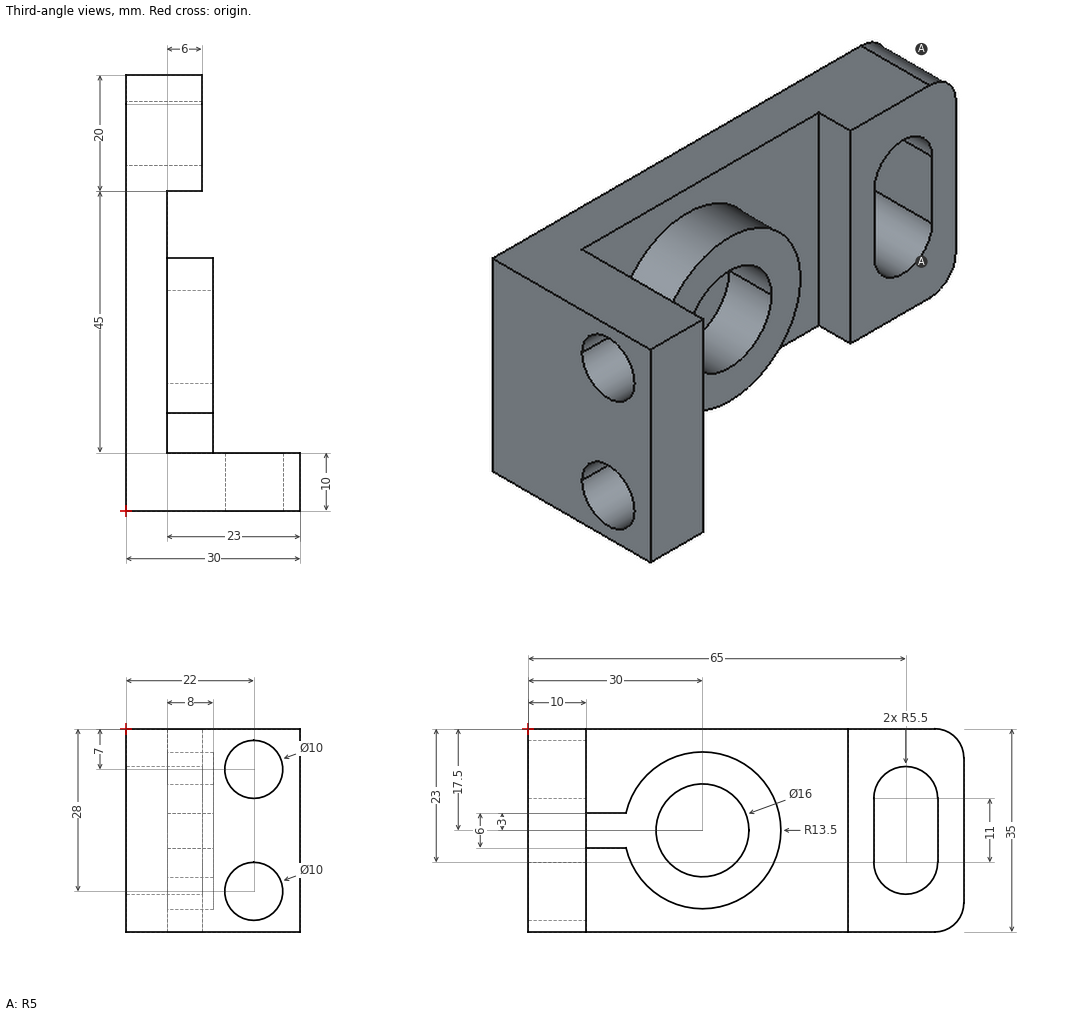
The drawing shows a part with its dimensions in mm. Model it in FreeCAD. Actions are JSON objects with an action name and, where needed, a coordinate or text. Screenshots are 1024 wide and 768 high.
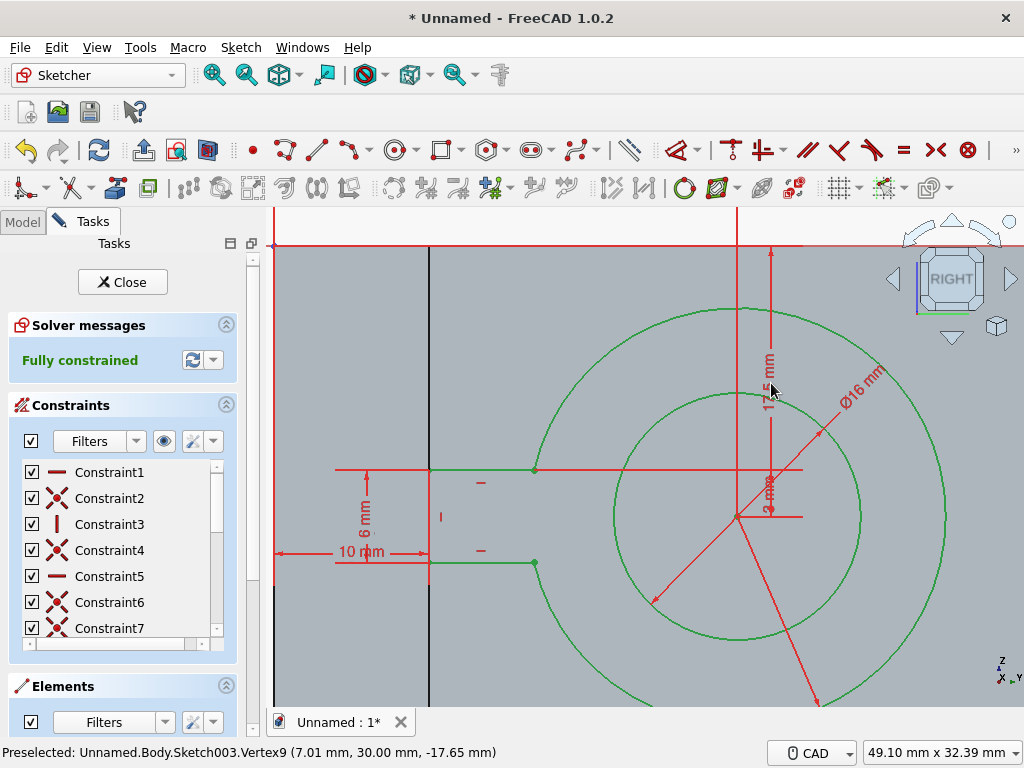
{"action": "left_click", "coordinate": [123, 282]}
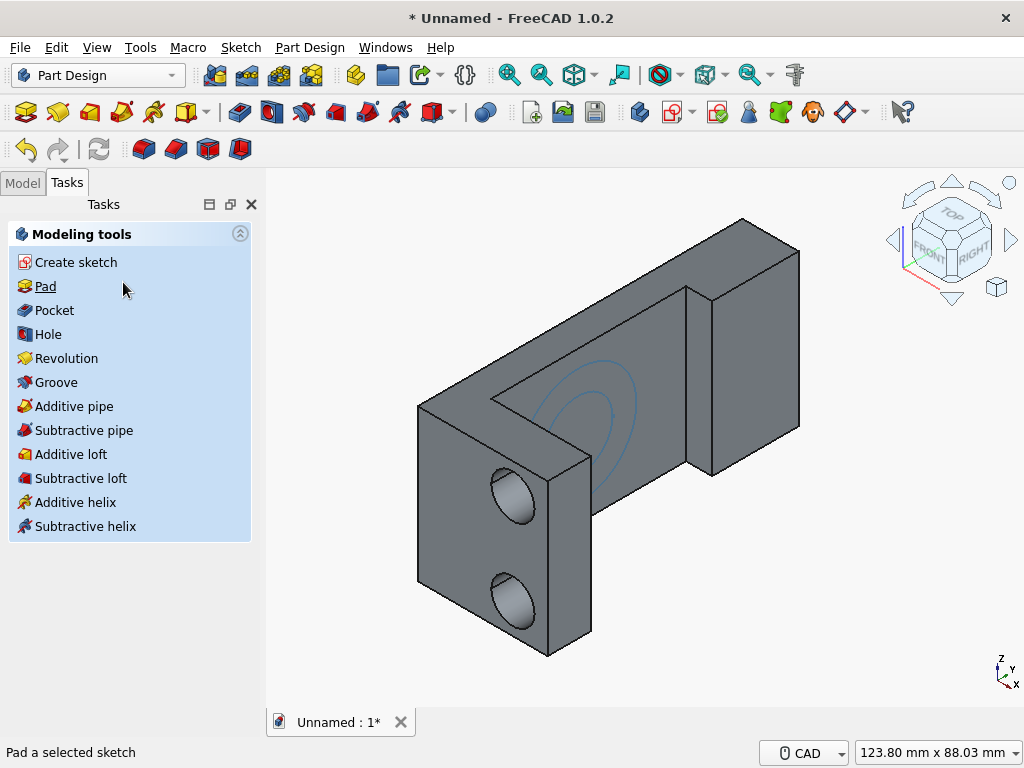
{"action": "left_click", "coordinate": [26, 112]}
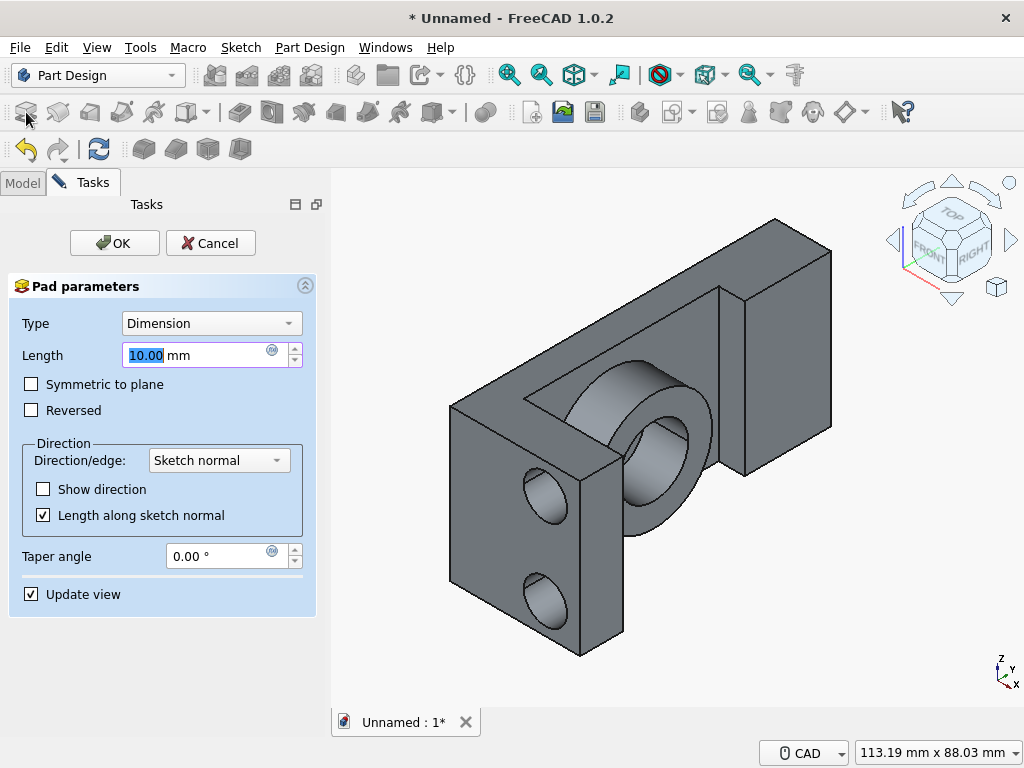
{"action": "type", "text": "8"}
{"action": "key", "text": "Tab"}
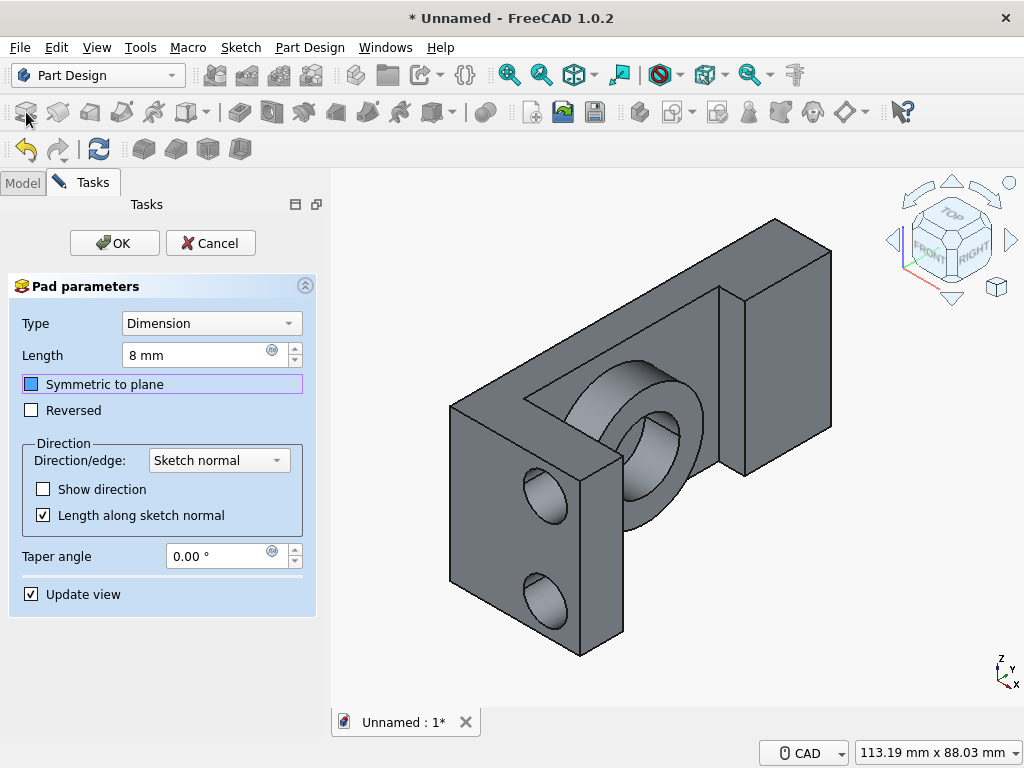
{"action": "left_click", "coordinate": [115, 243]}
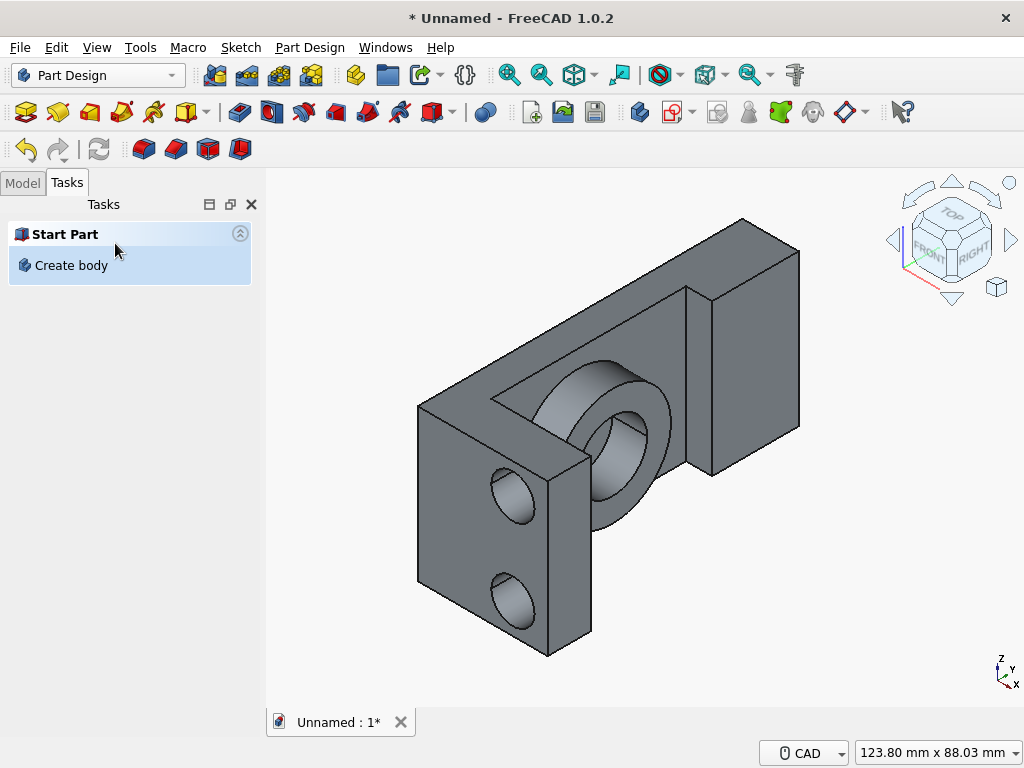
{"action": "key", "text": "2"}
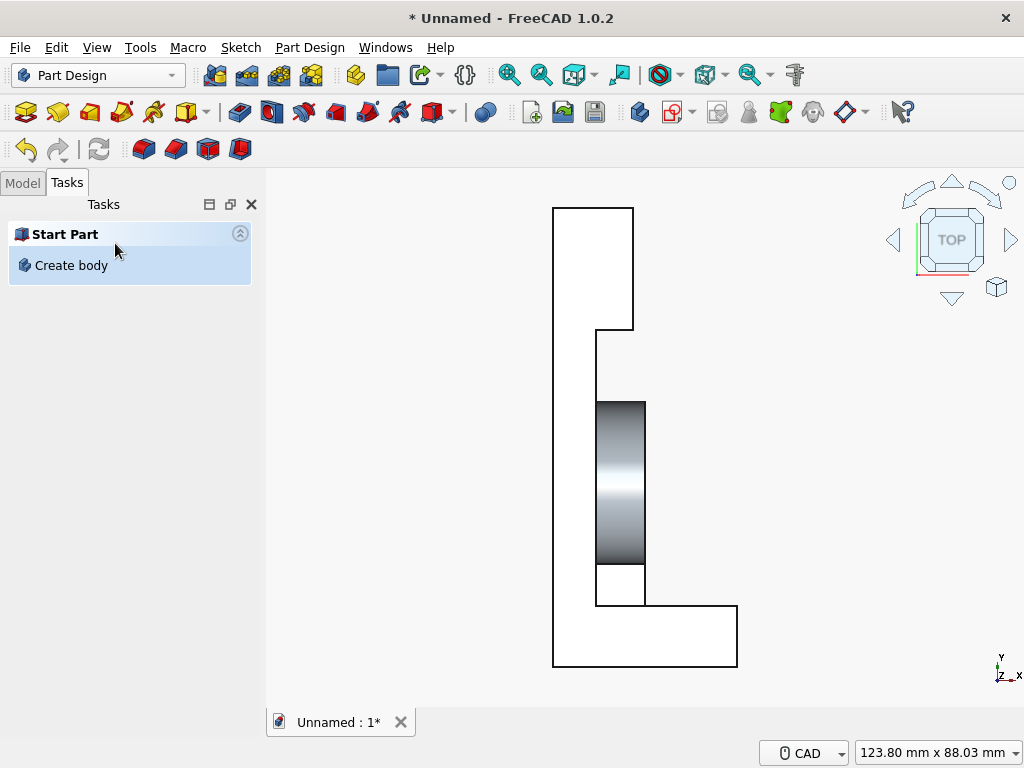
{"action": "left_click", "coordinate": [593, 207]}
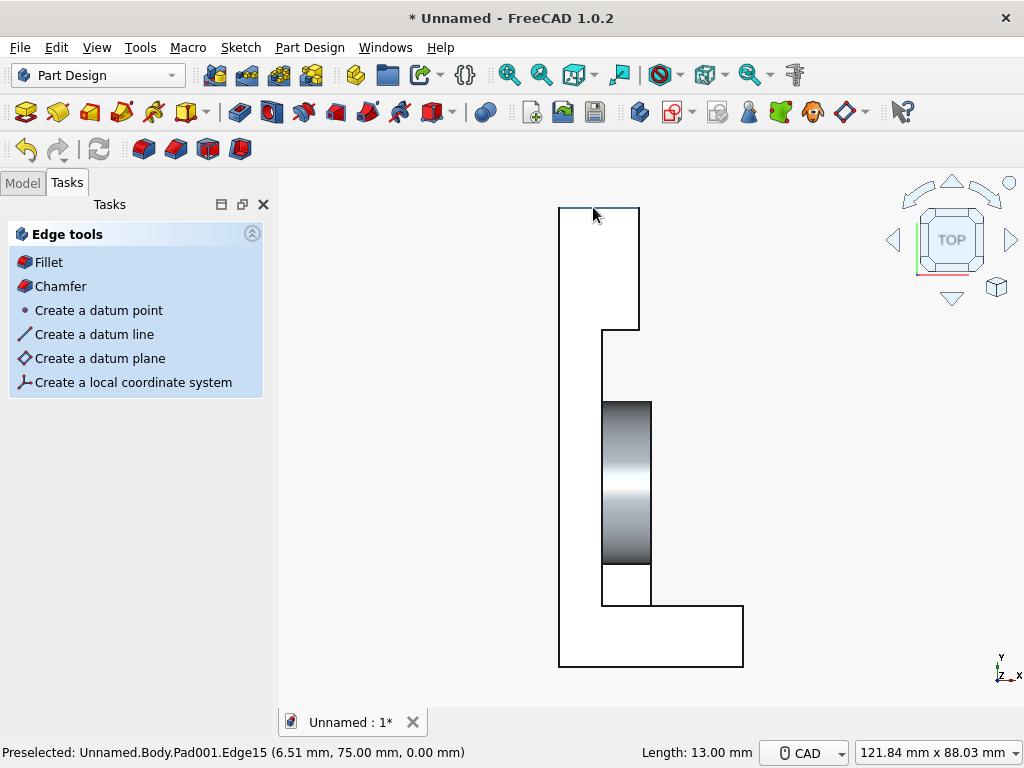
{"action": "key", "text": "0"}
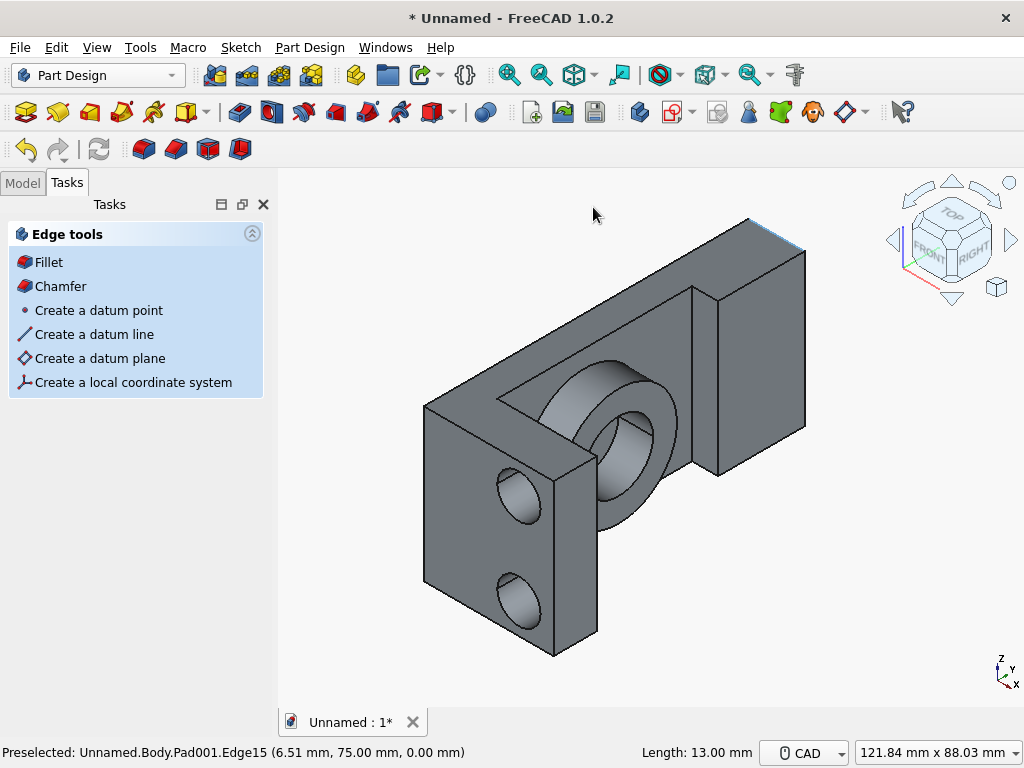
{"action": "key", "text": "1"}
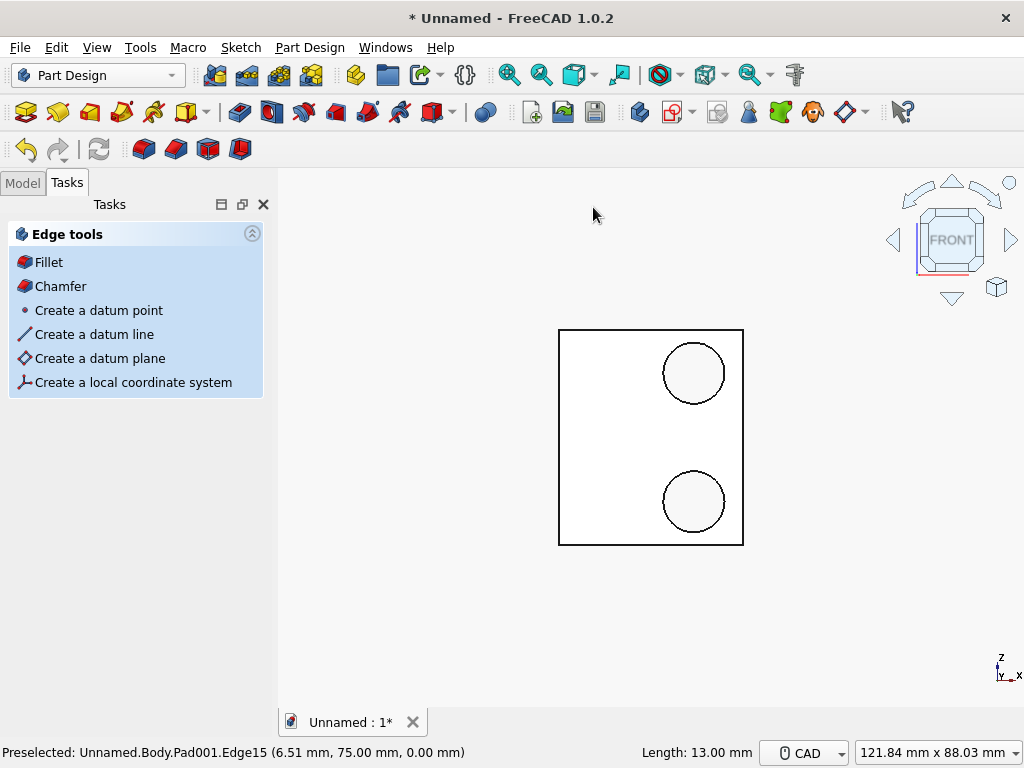
{"action": "left_click", "coordinate": [510, 76]}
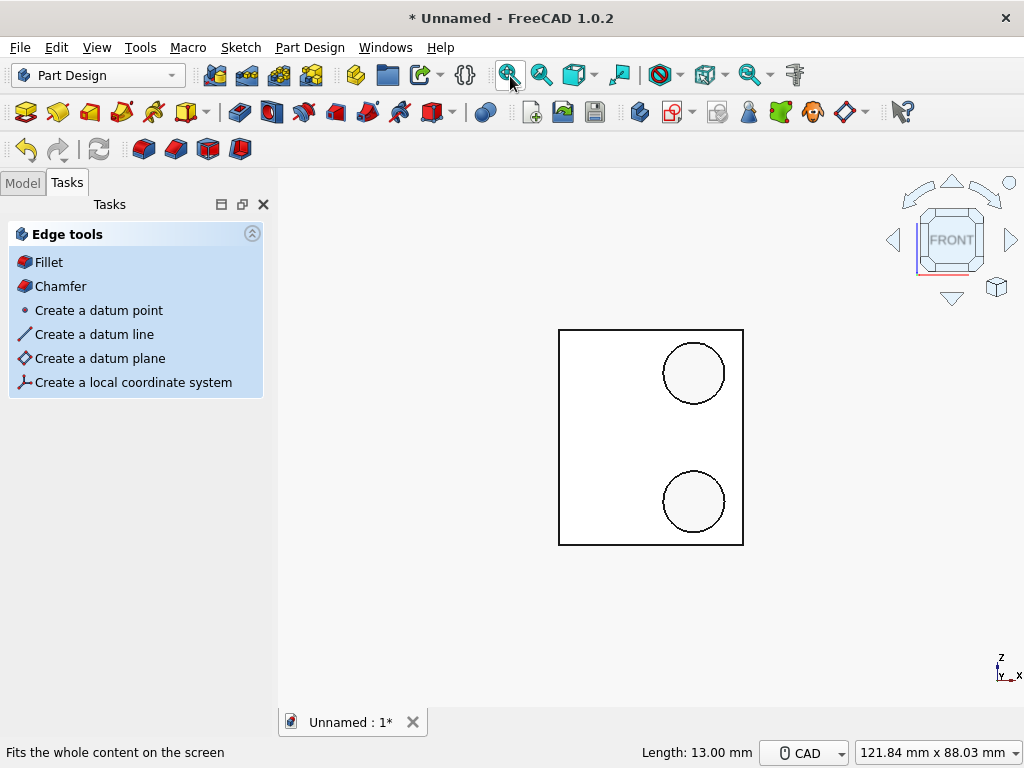
{"action": "key", "text": "3"}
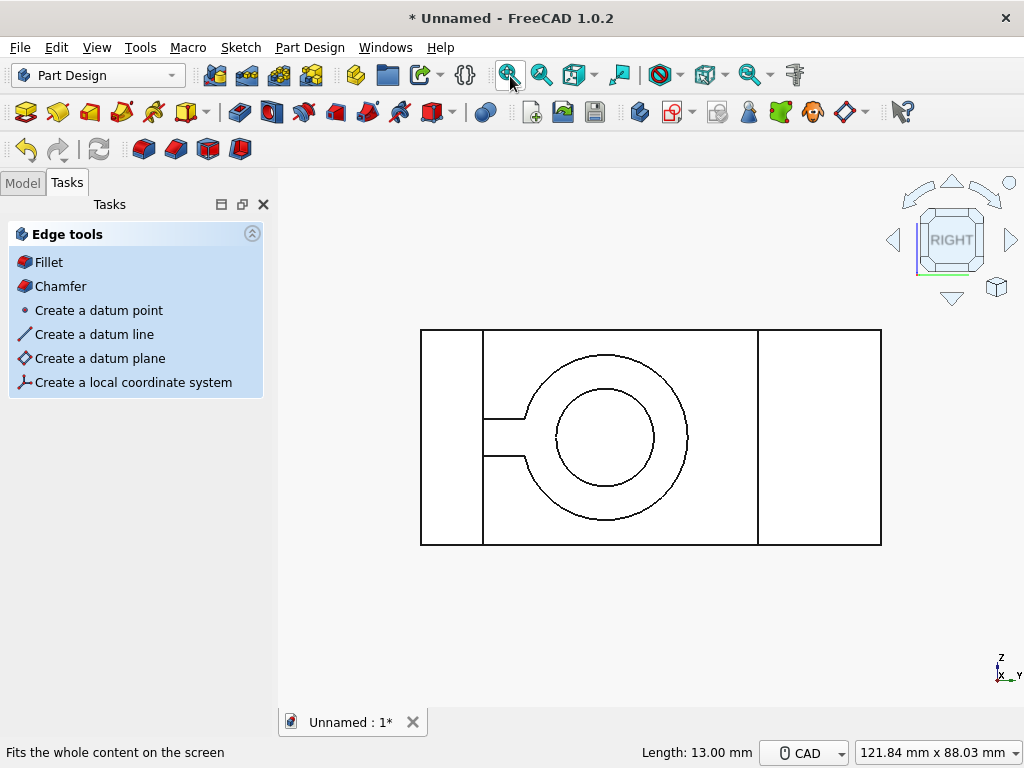
{"action": "key", "text": "5"}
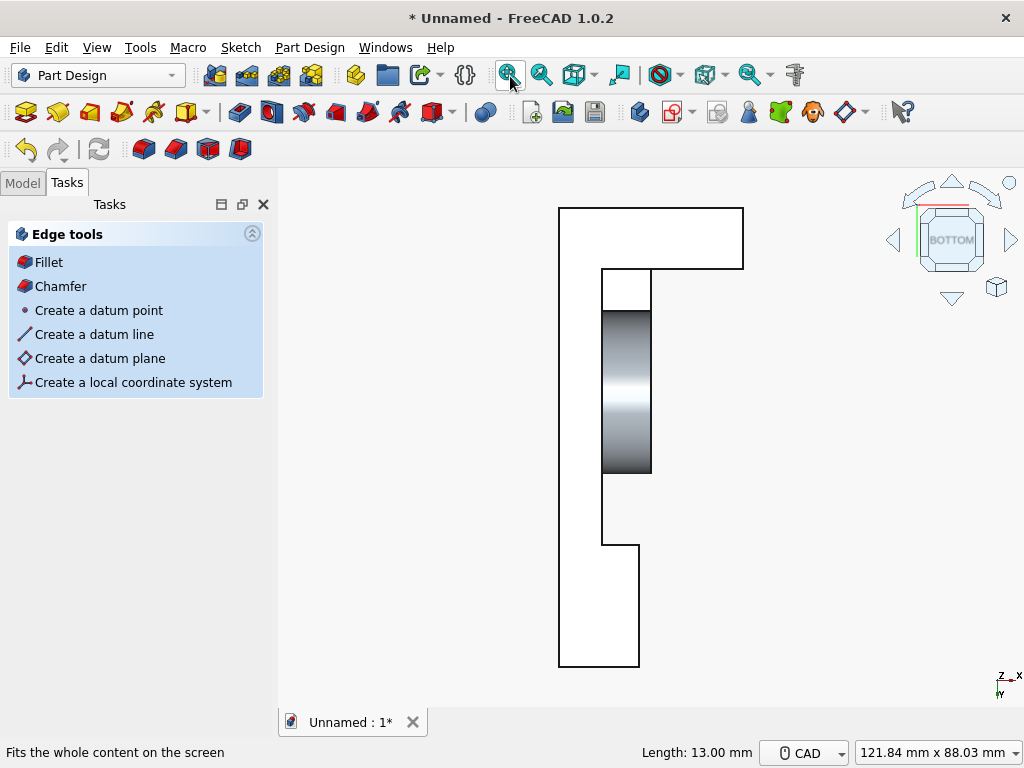
{"action": "left_click", "coordinate": [599, 666], "text": "ctrl"}